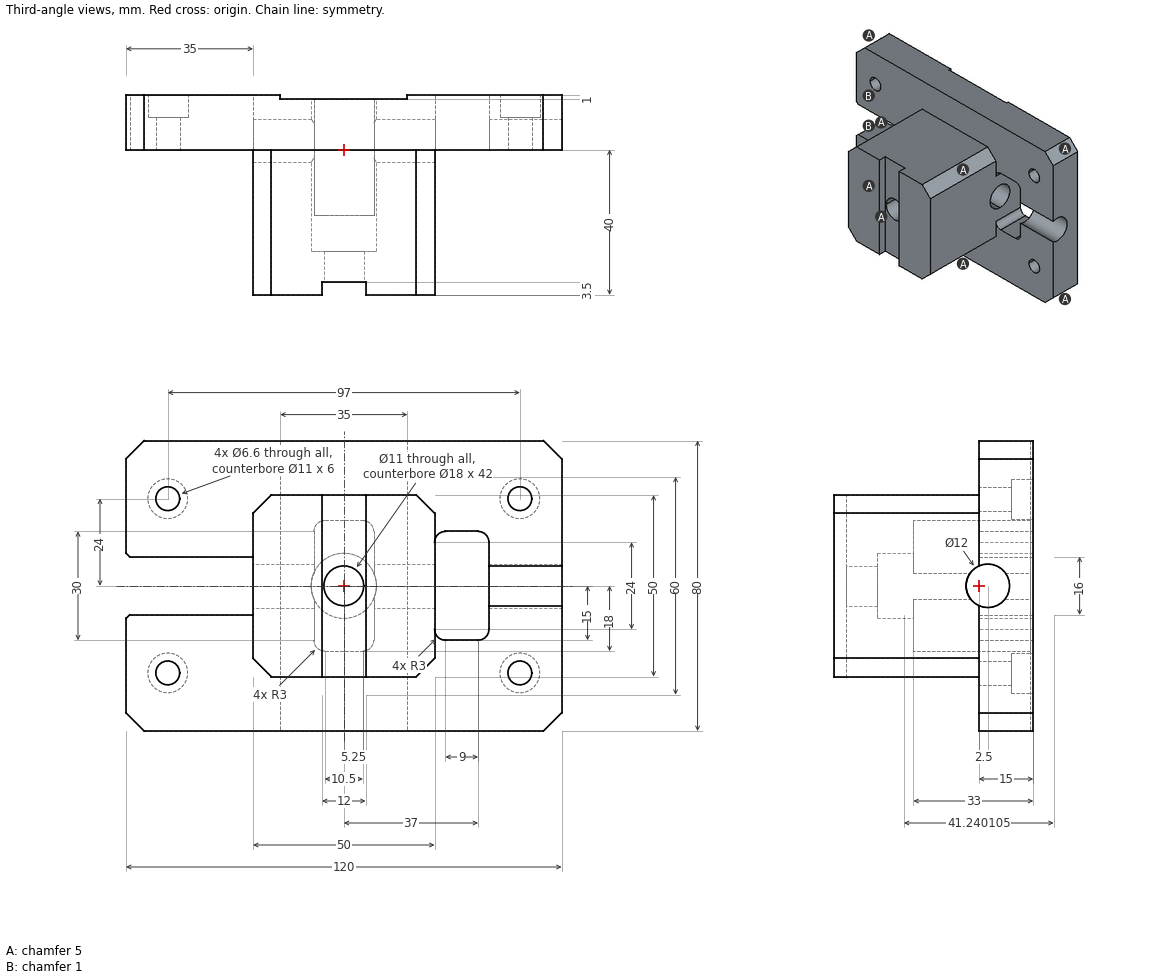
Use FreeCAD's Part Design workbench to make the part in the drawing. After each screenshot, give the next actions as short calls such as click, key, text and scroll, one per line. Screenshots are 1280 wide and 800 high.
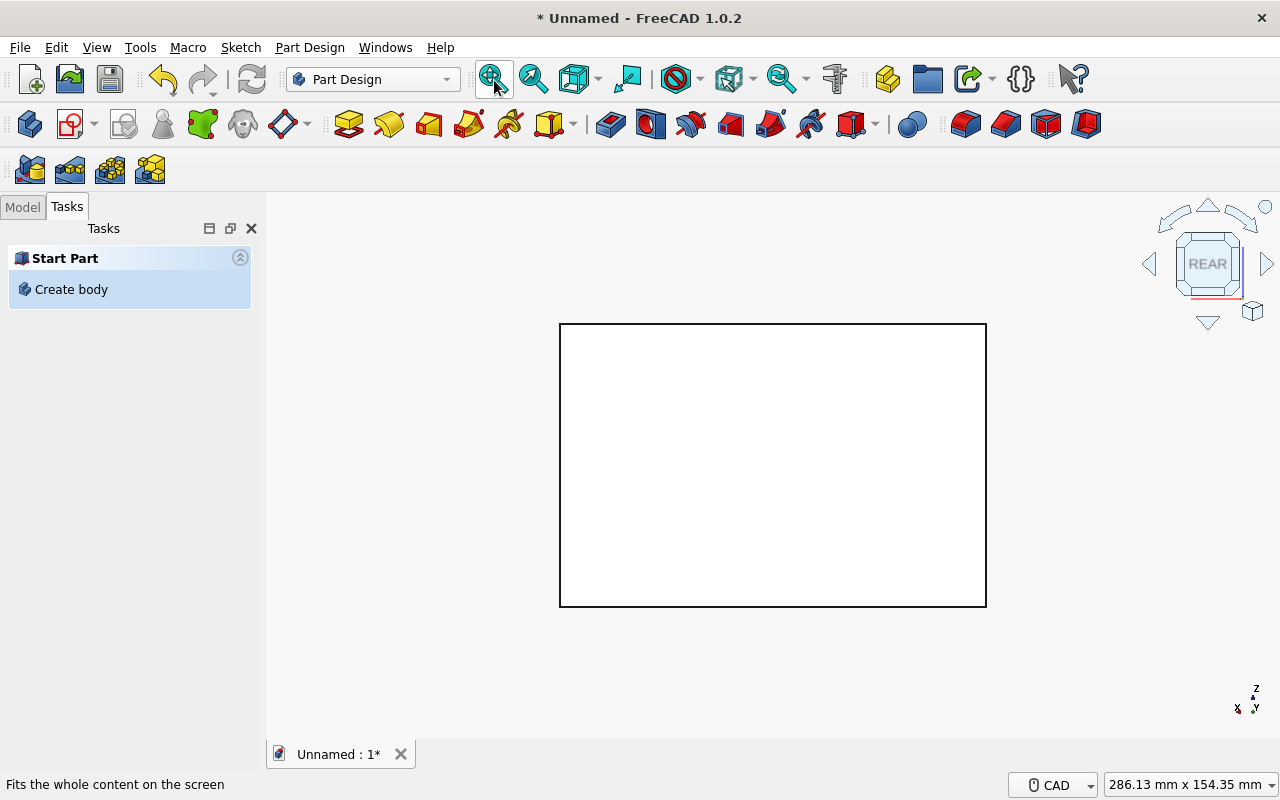
click(712, 465)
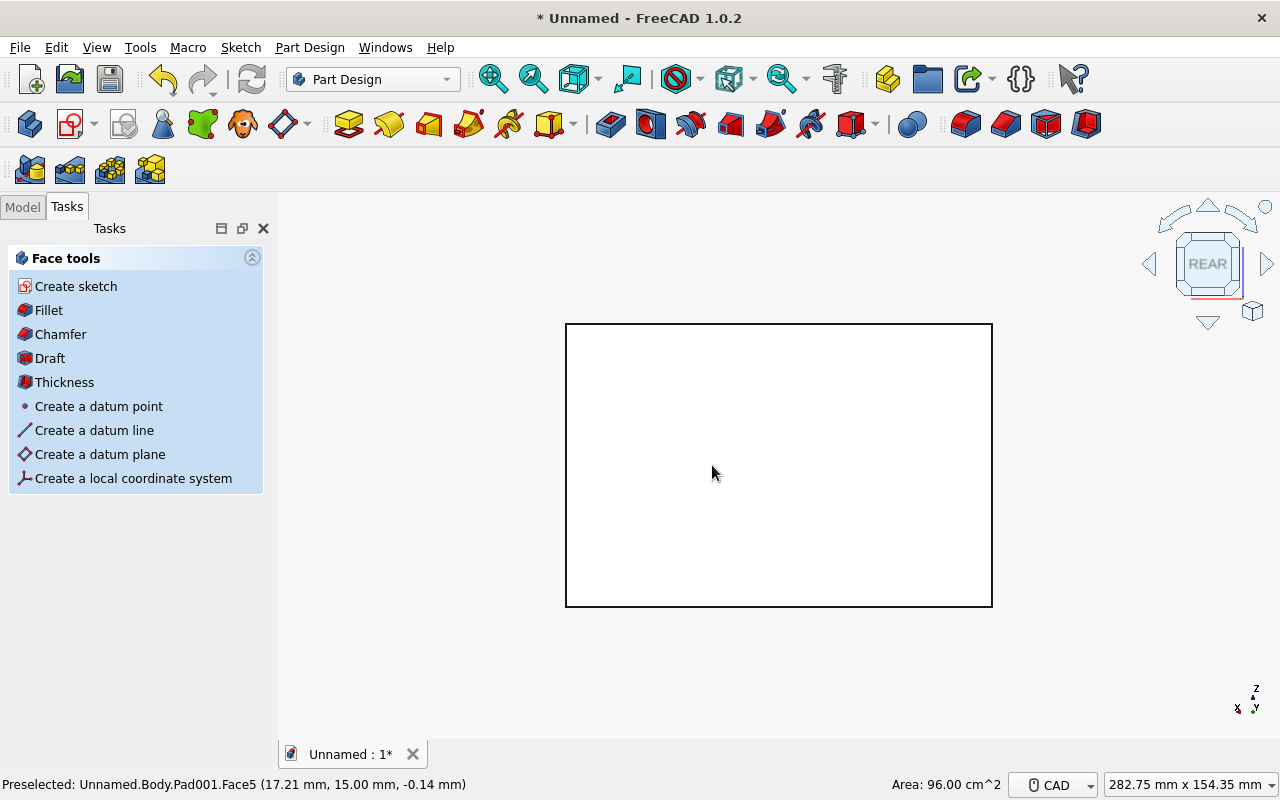
click(70, 124)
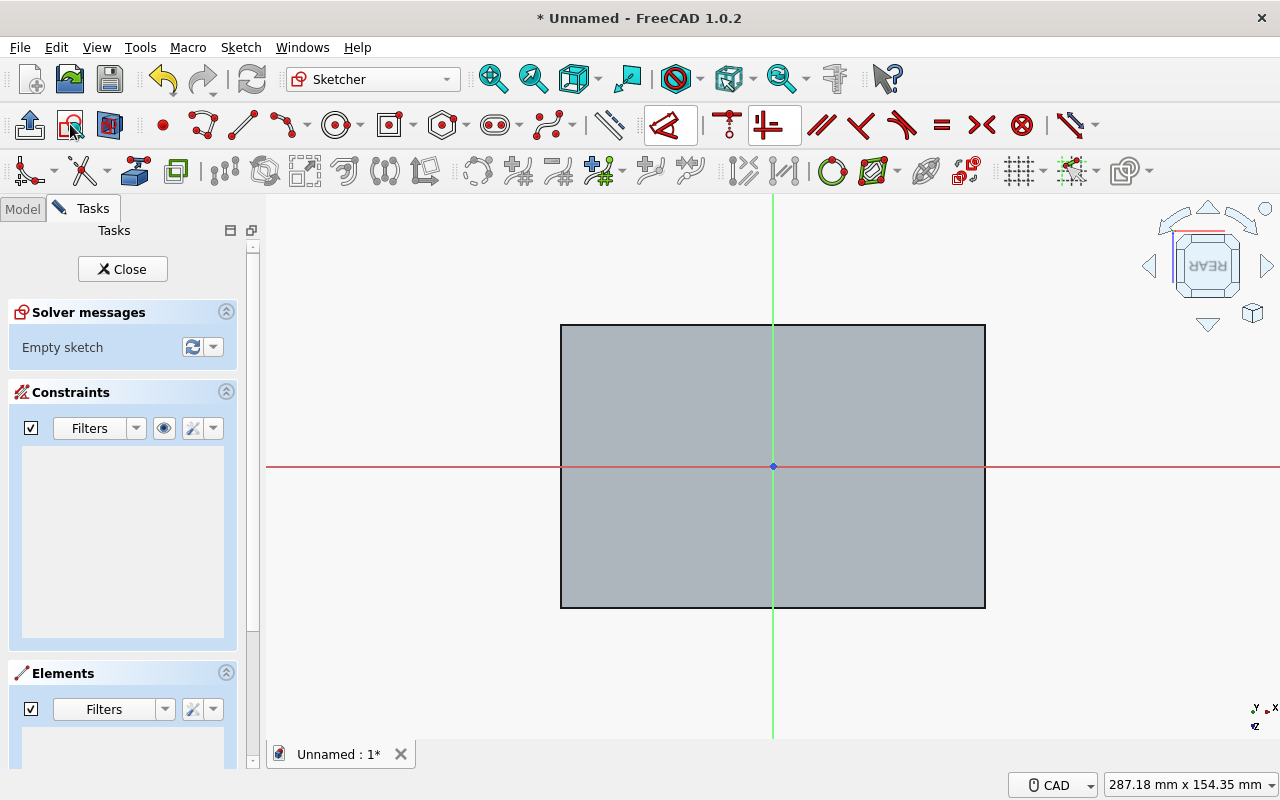
scroll(813, 466, up, 5)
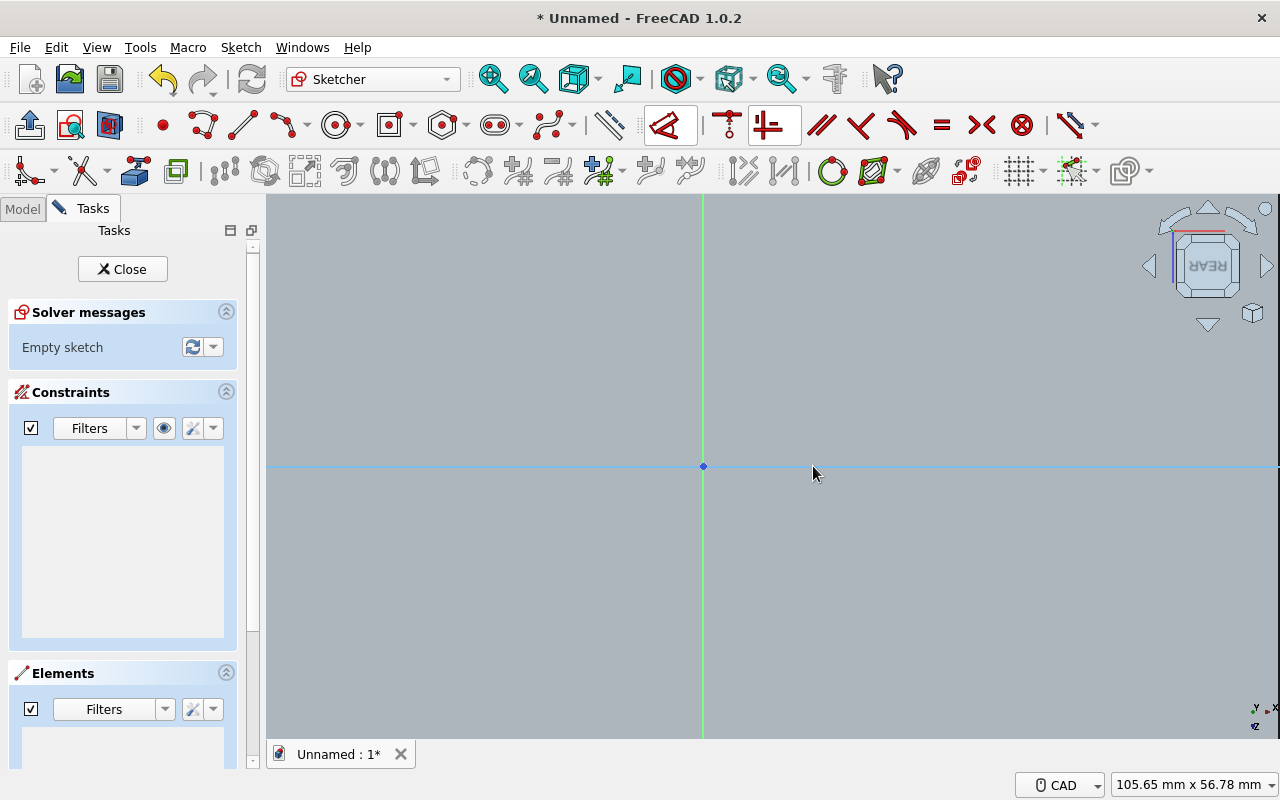
click(244, 126)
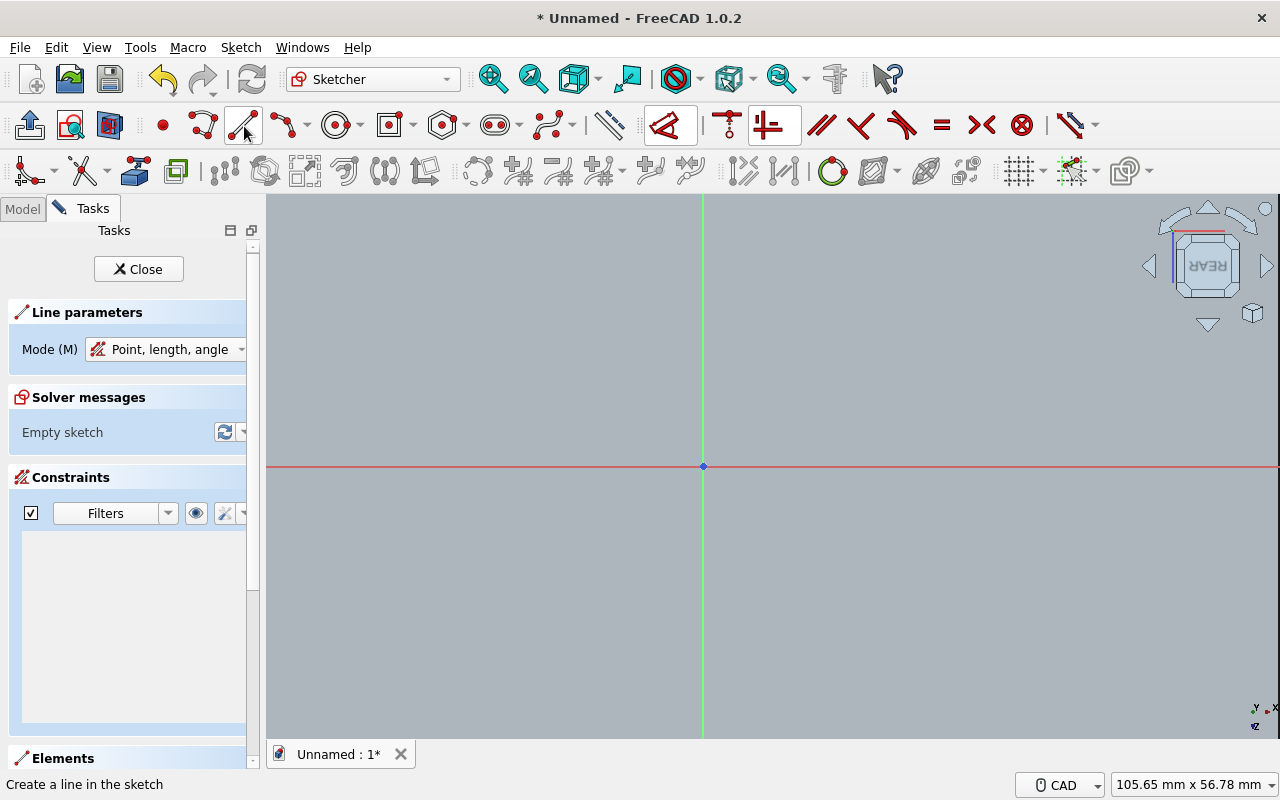
click(754, 294)
click(653, 294)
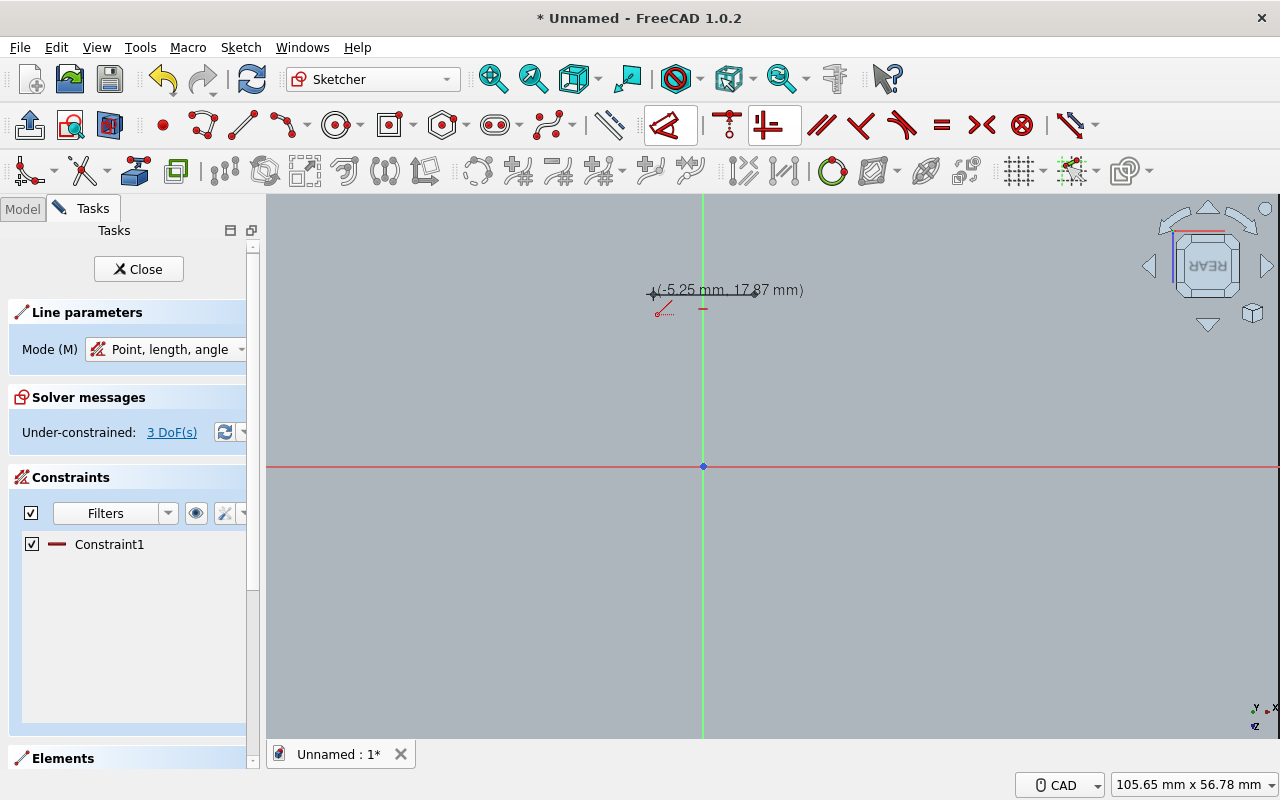
click(624, 323)
click(624, 610)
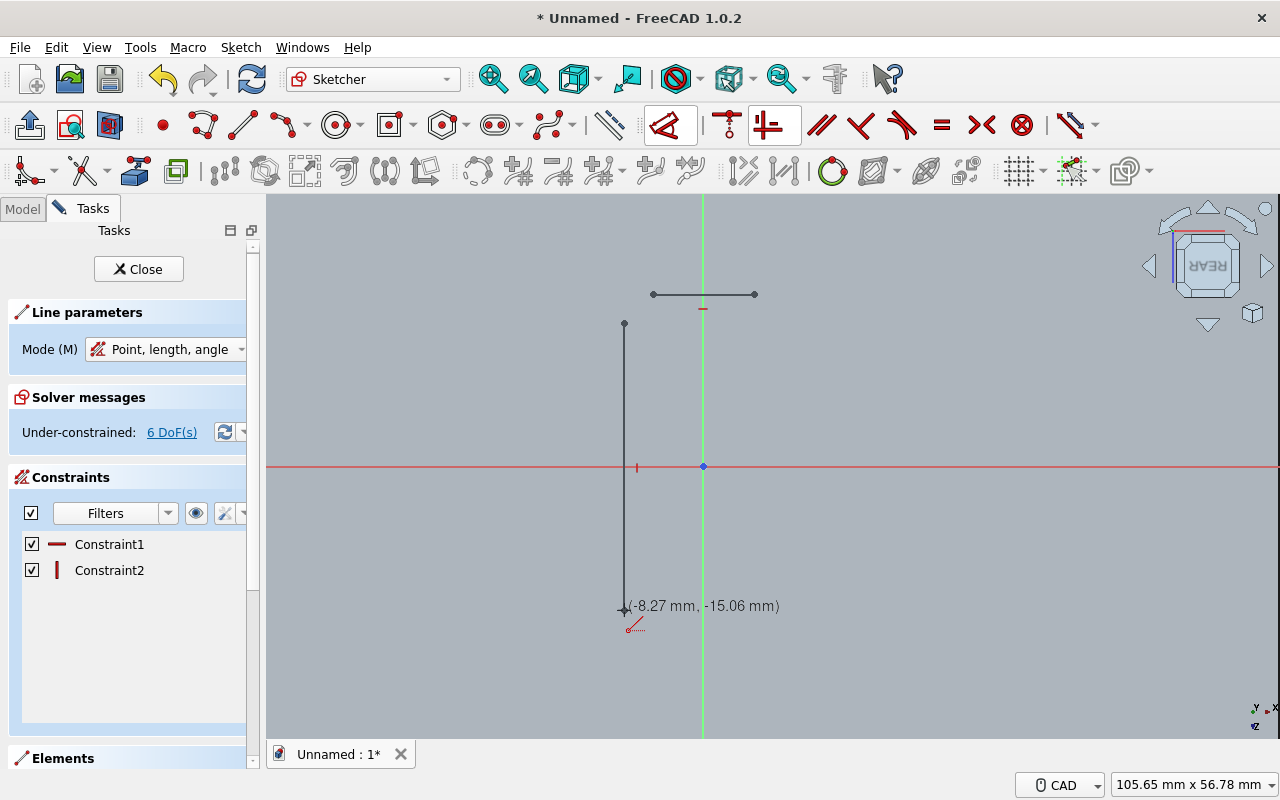
click(653, 639)
click(754, 639)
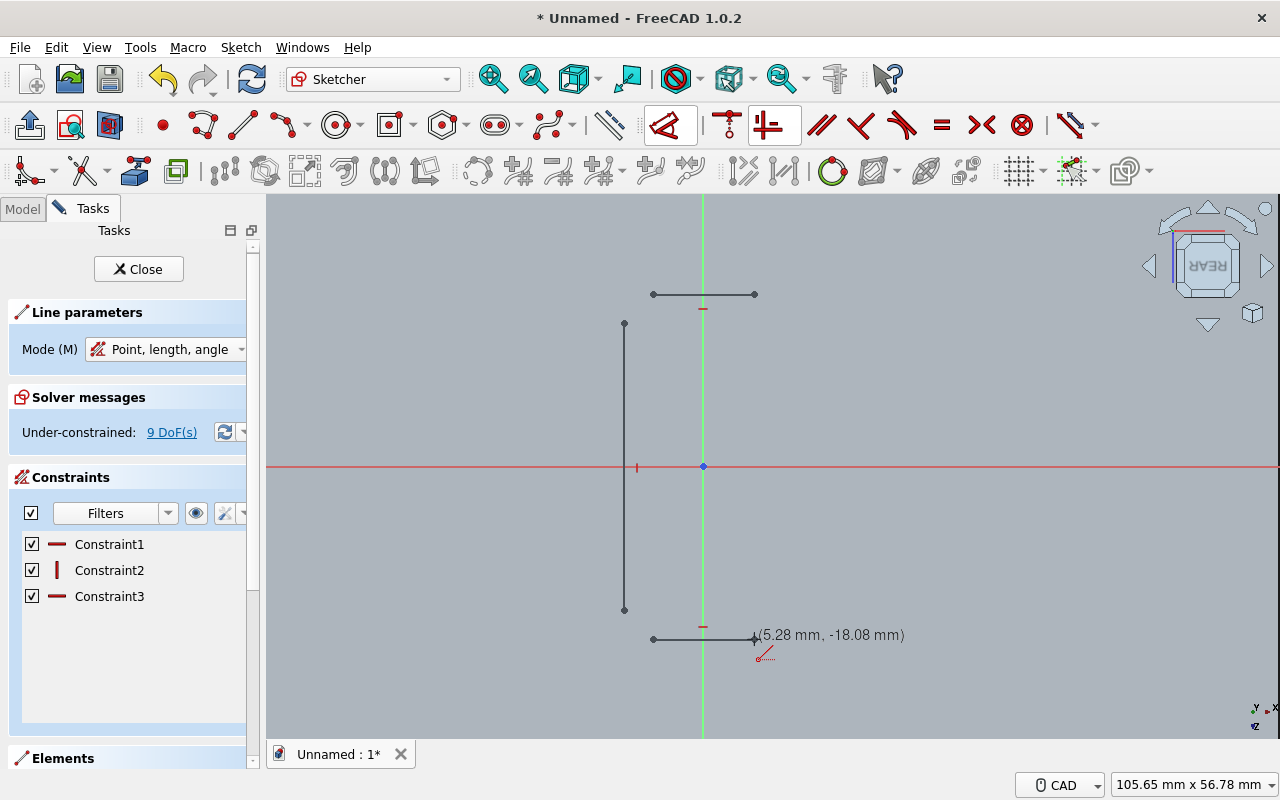
click(783, 610)
click(783, 323)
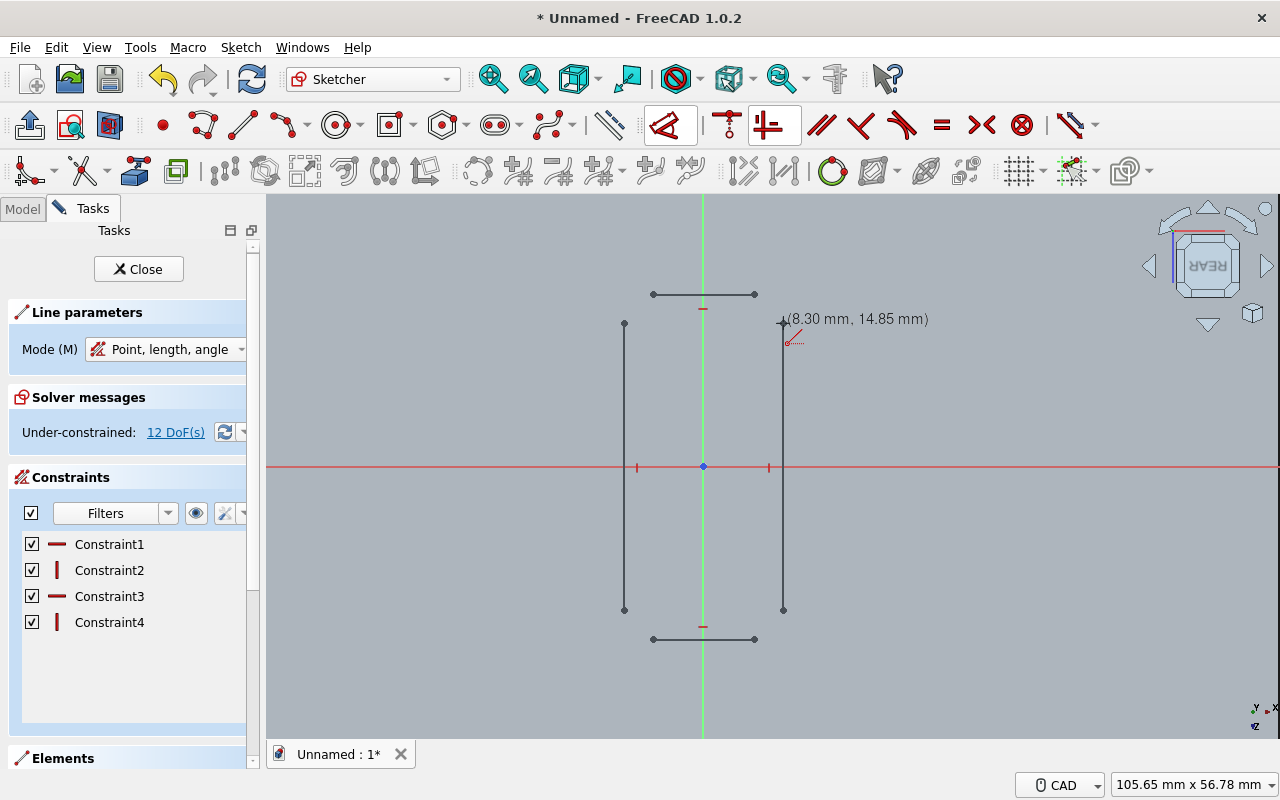
click(284, 126)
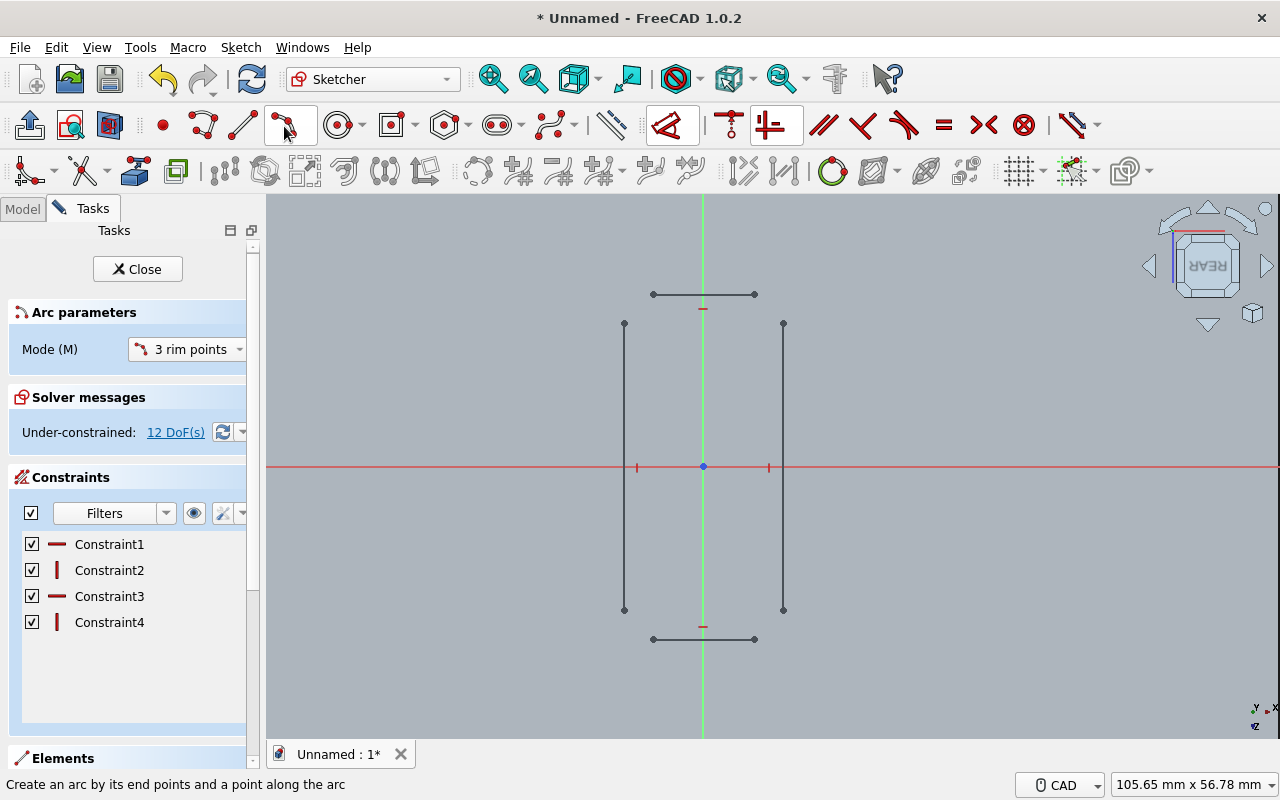
click(653, 295)
click(624, 324)